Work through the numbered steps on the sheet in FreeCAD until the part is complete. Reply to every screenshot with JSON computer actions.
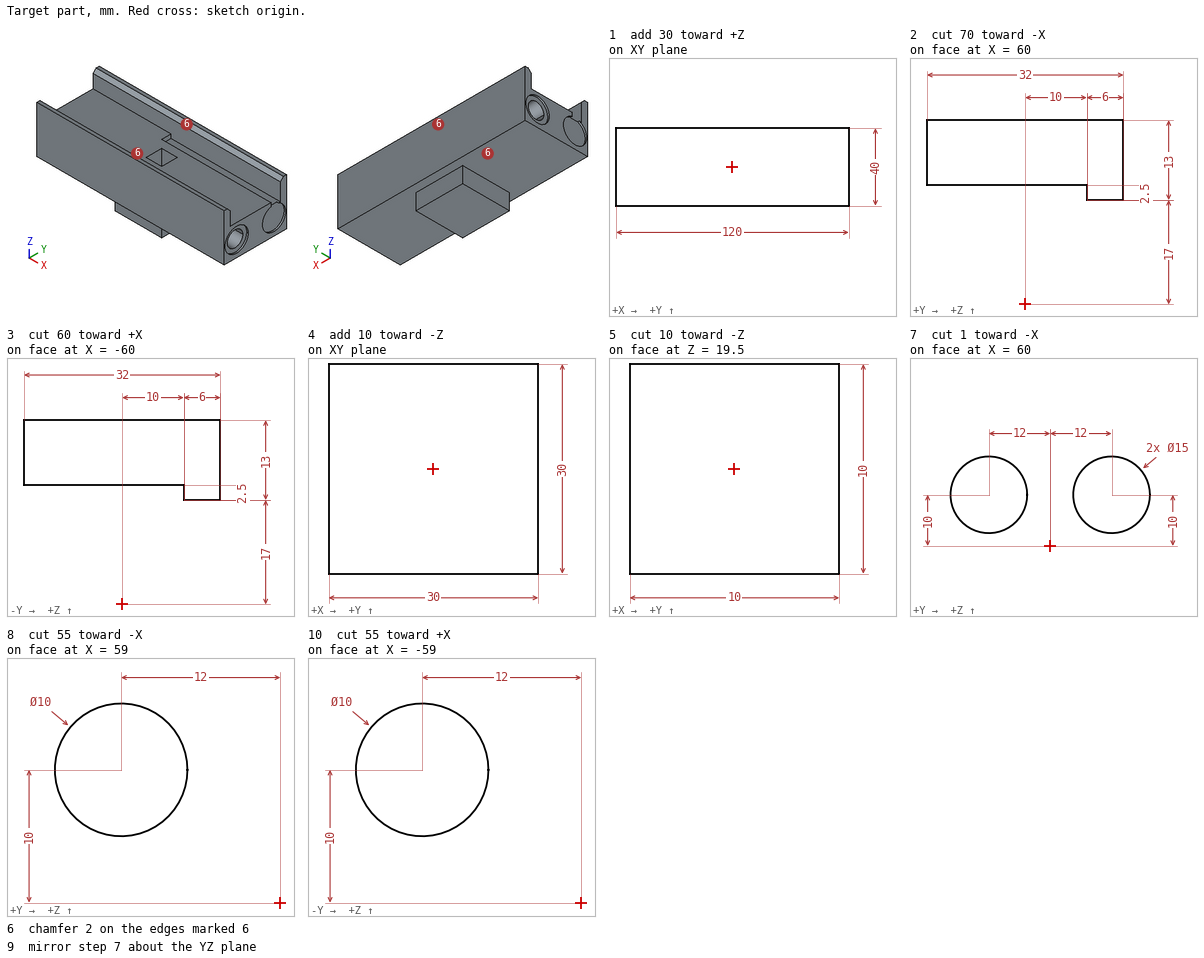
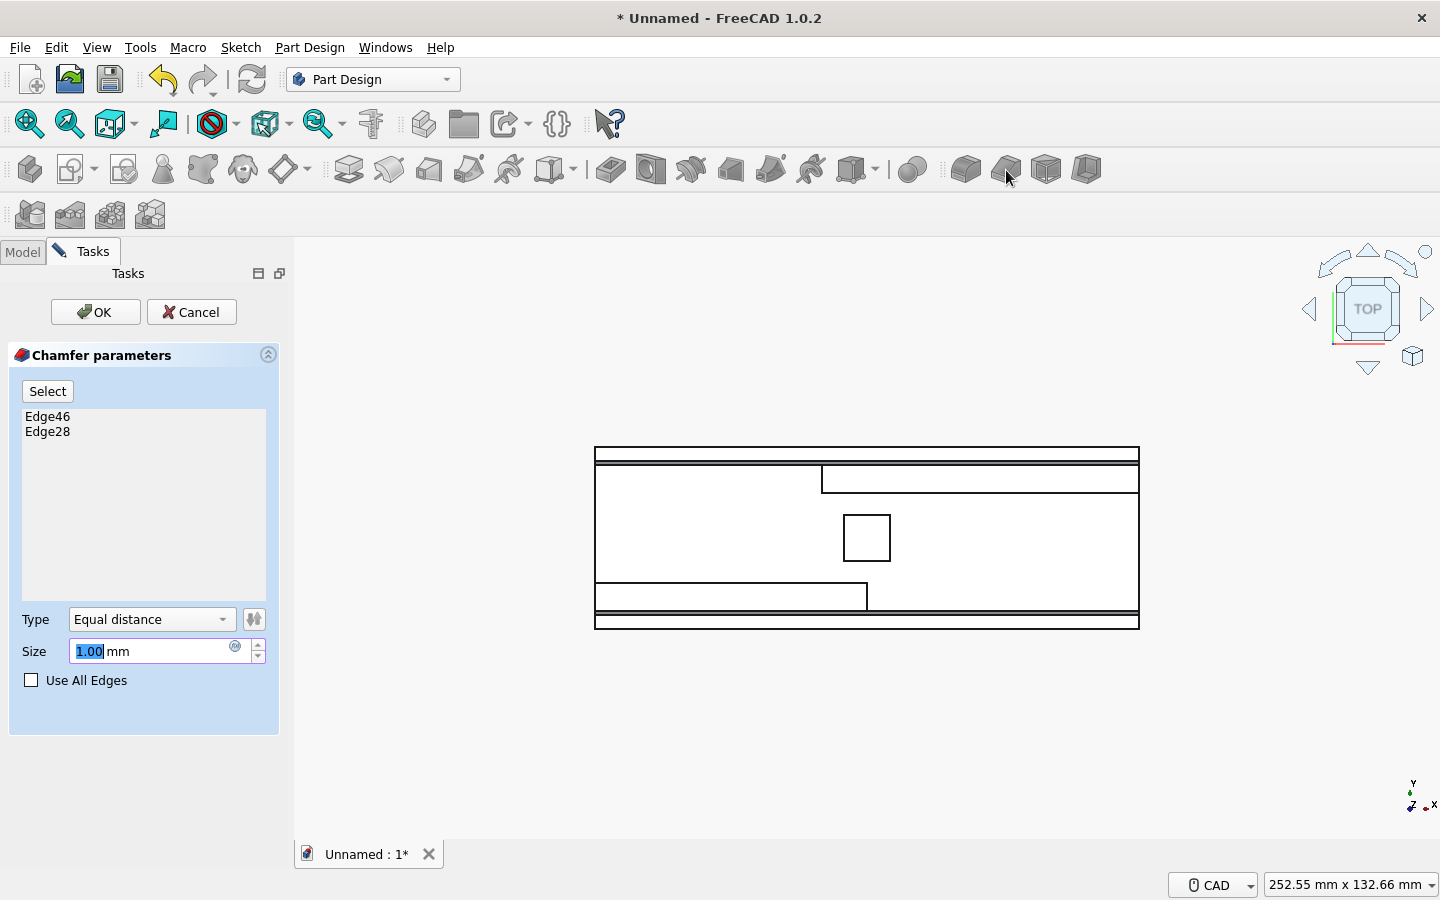
{"action": "type", "text": "2"}
{"action": "key", "text": "Tab"}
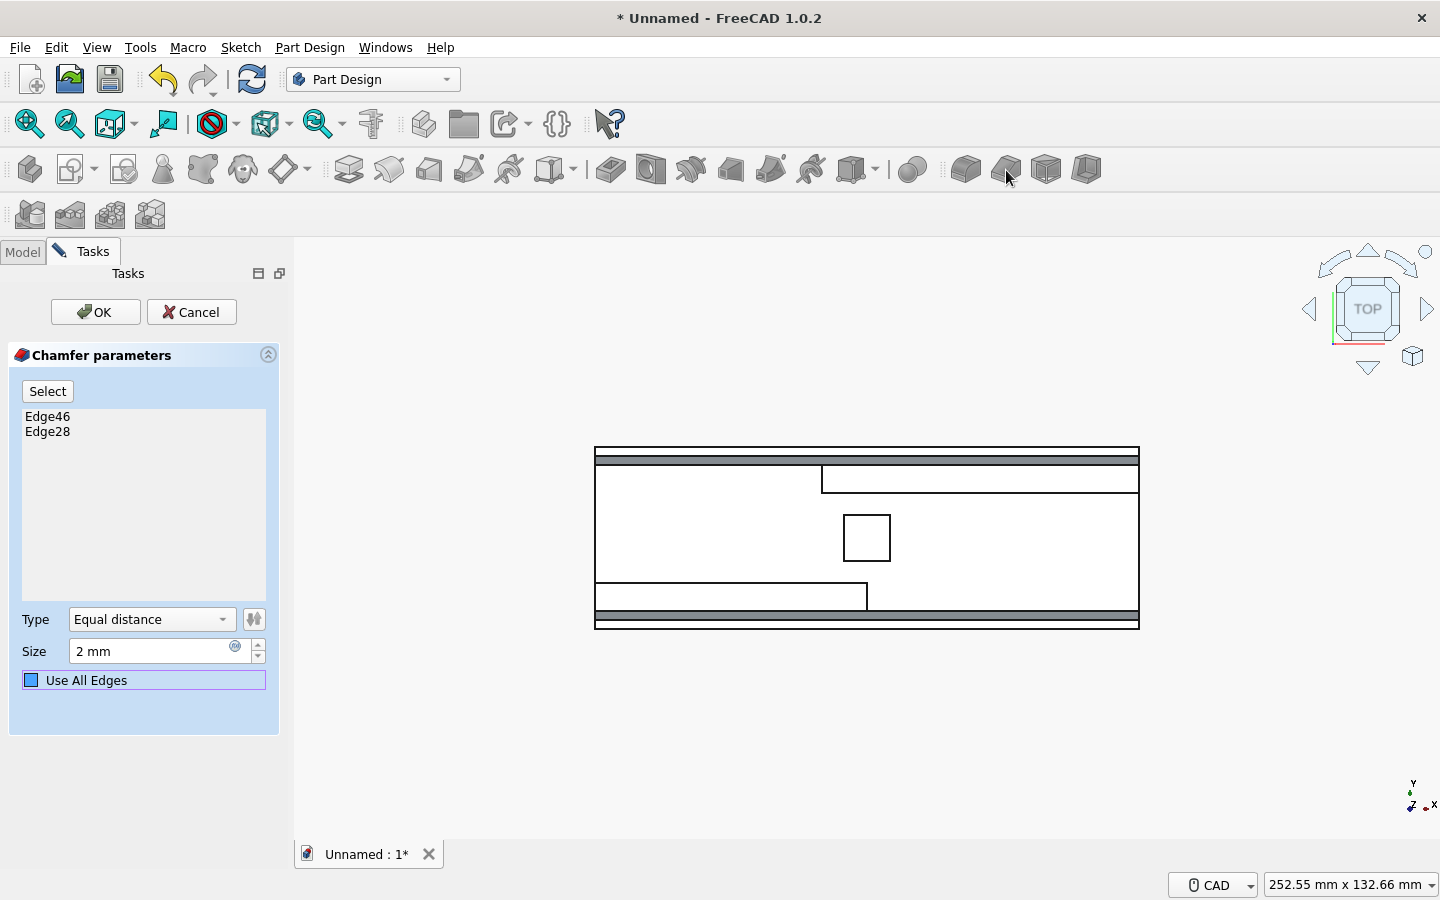
{"action": "left_click", "coordinate": [96, 312]}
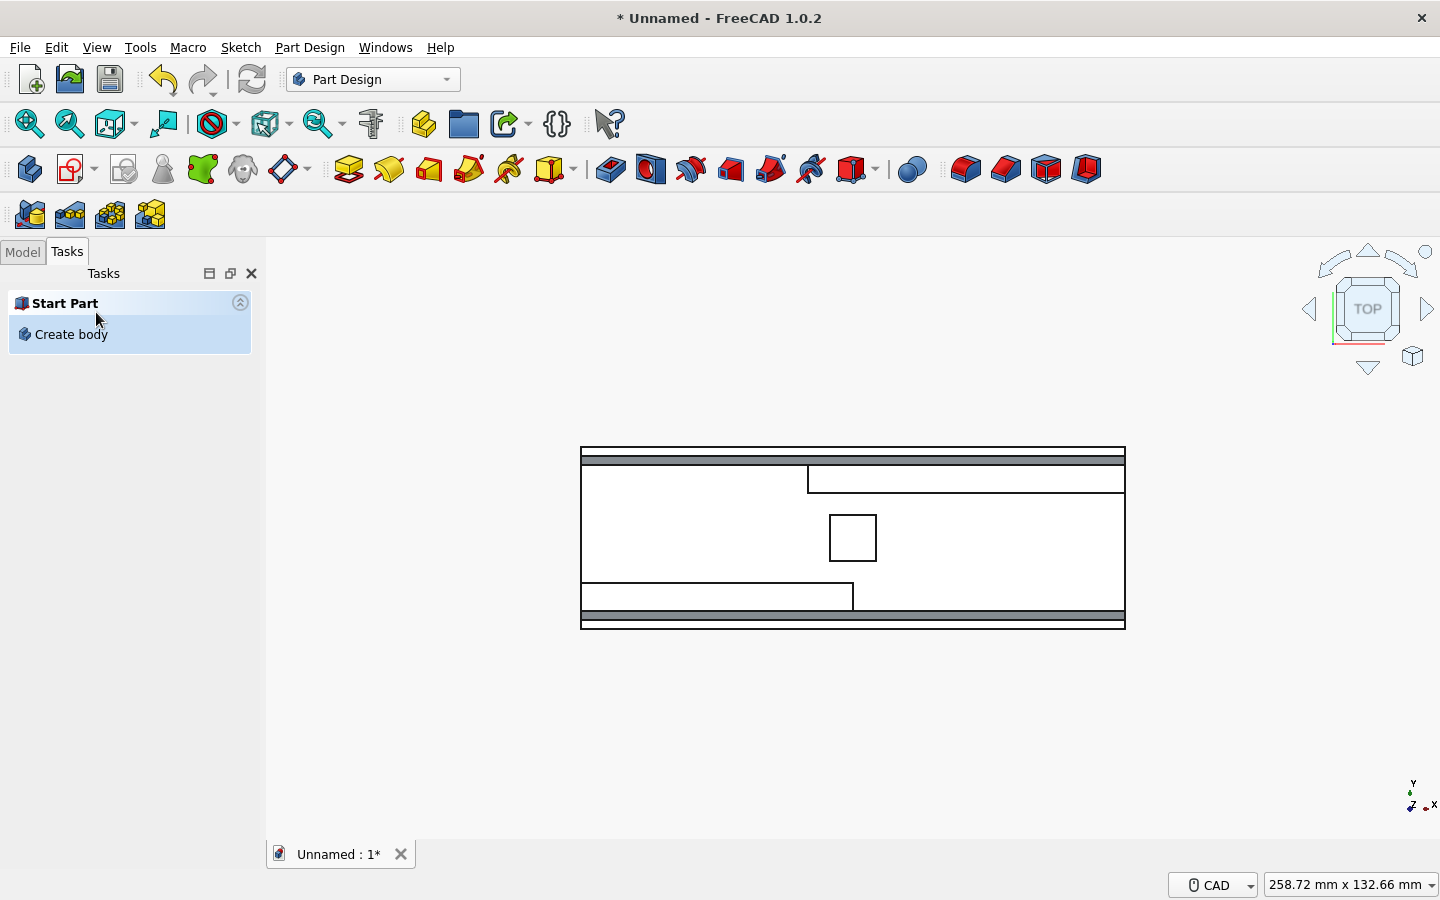
{"action": "key", "text": "0"}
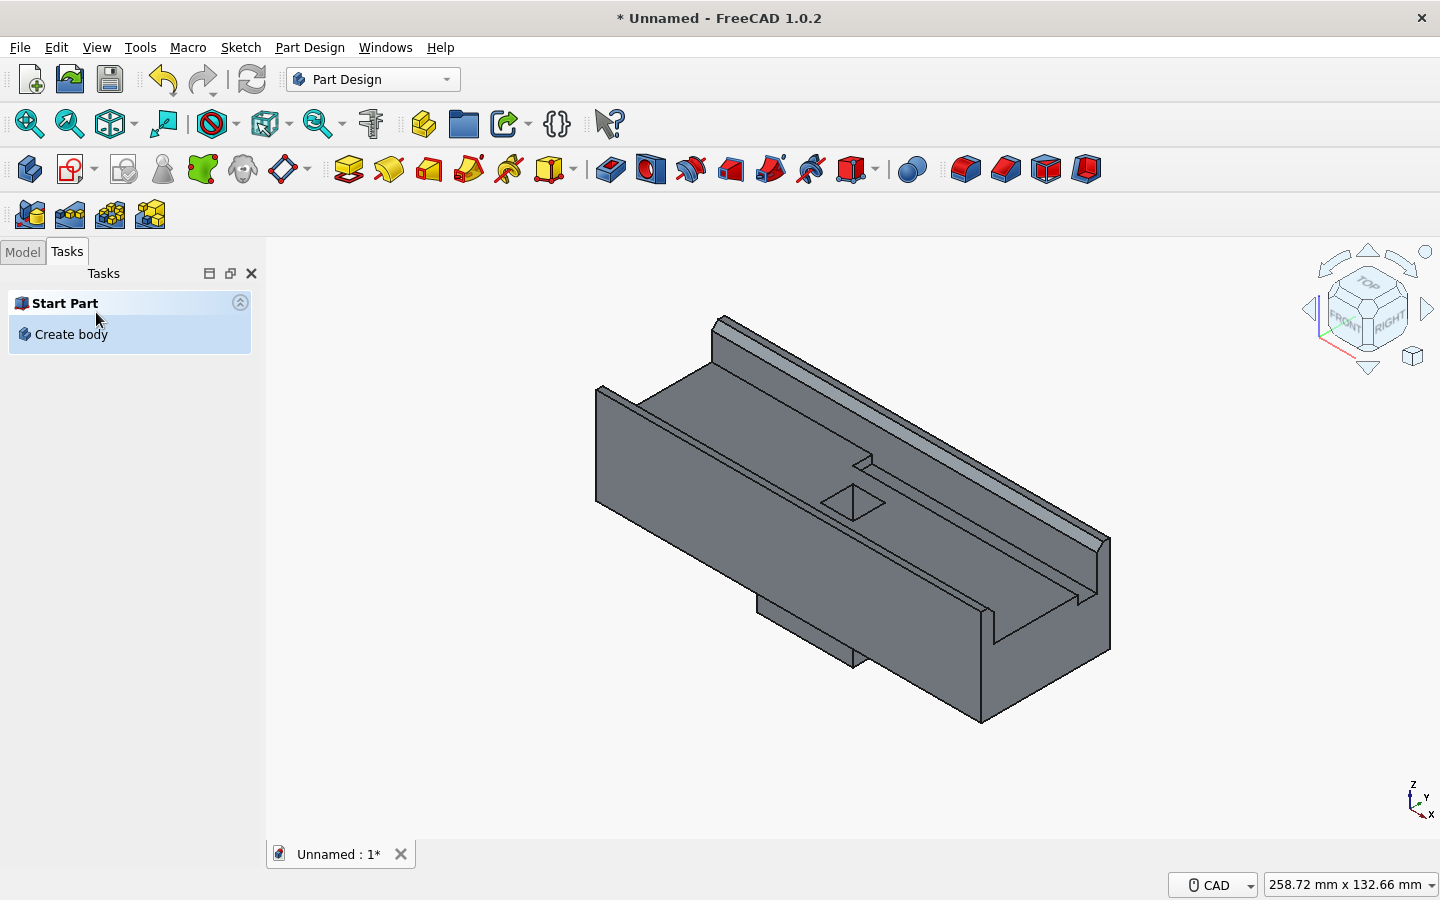
{"action": "left_click", "coordinate": [1046, 646]}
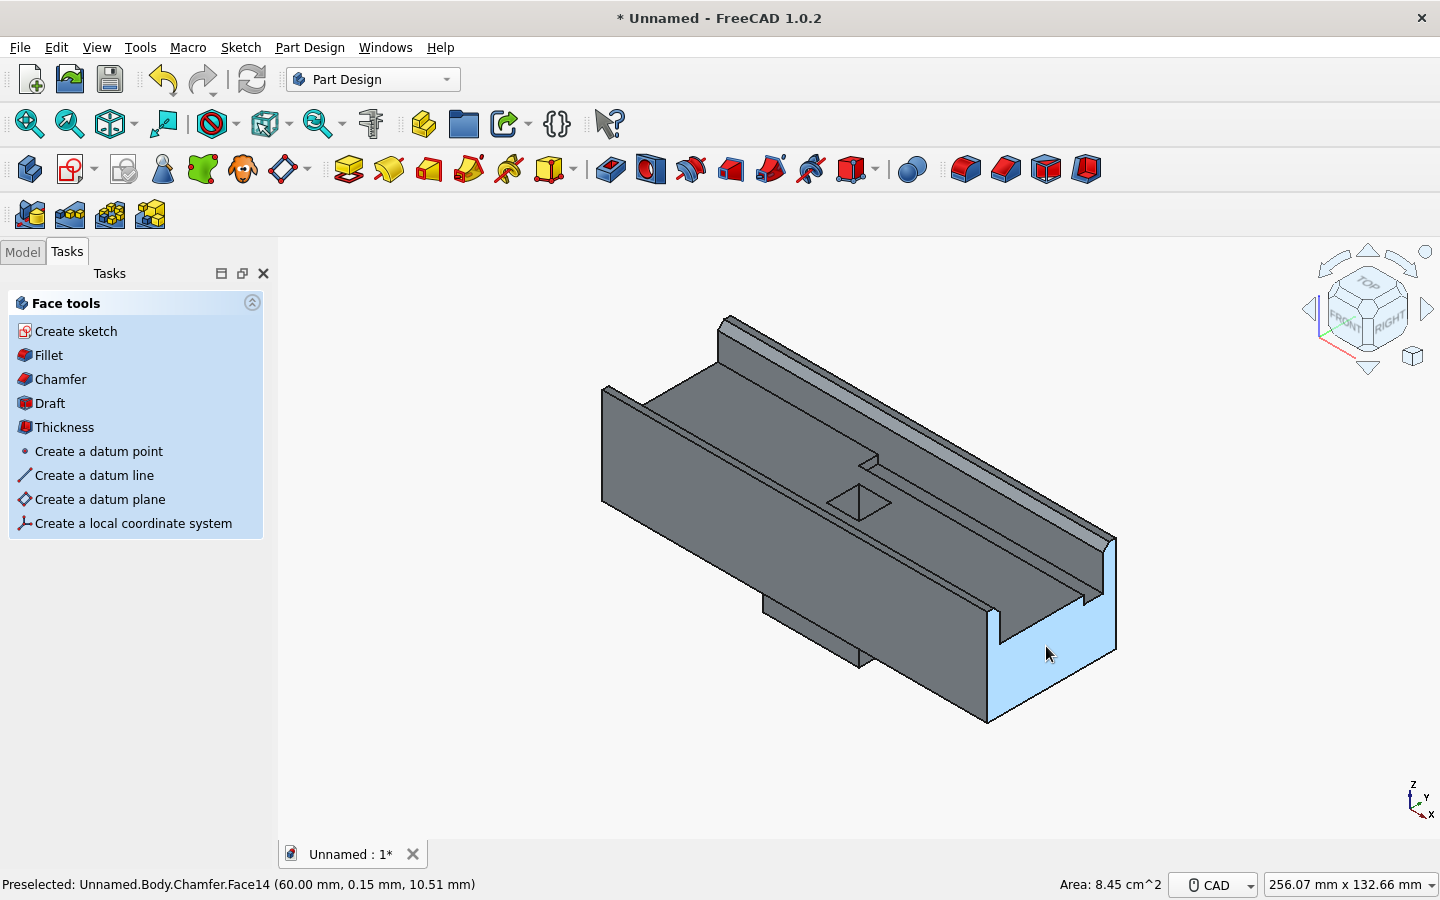
{"action": "left_click", "coordinate": [70, 170]}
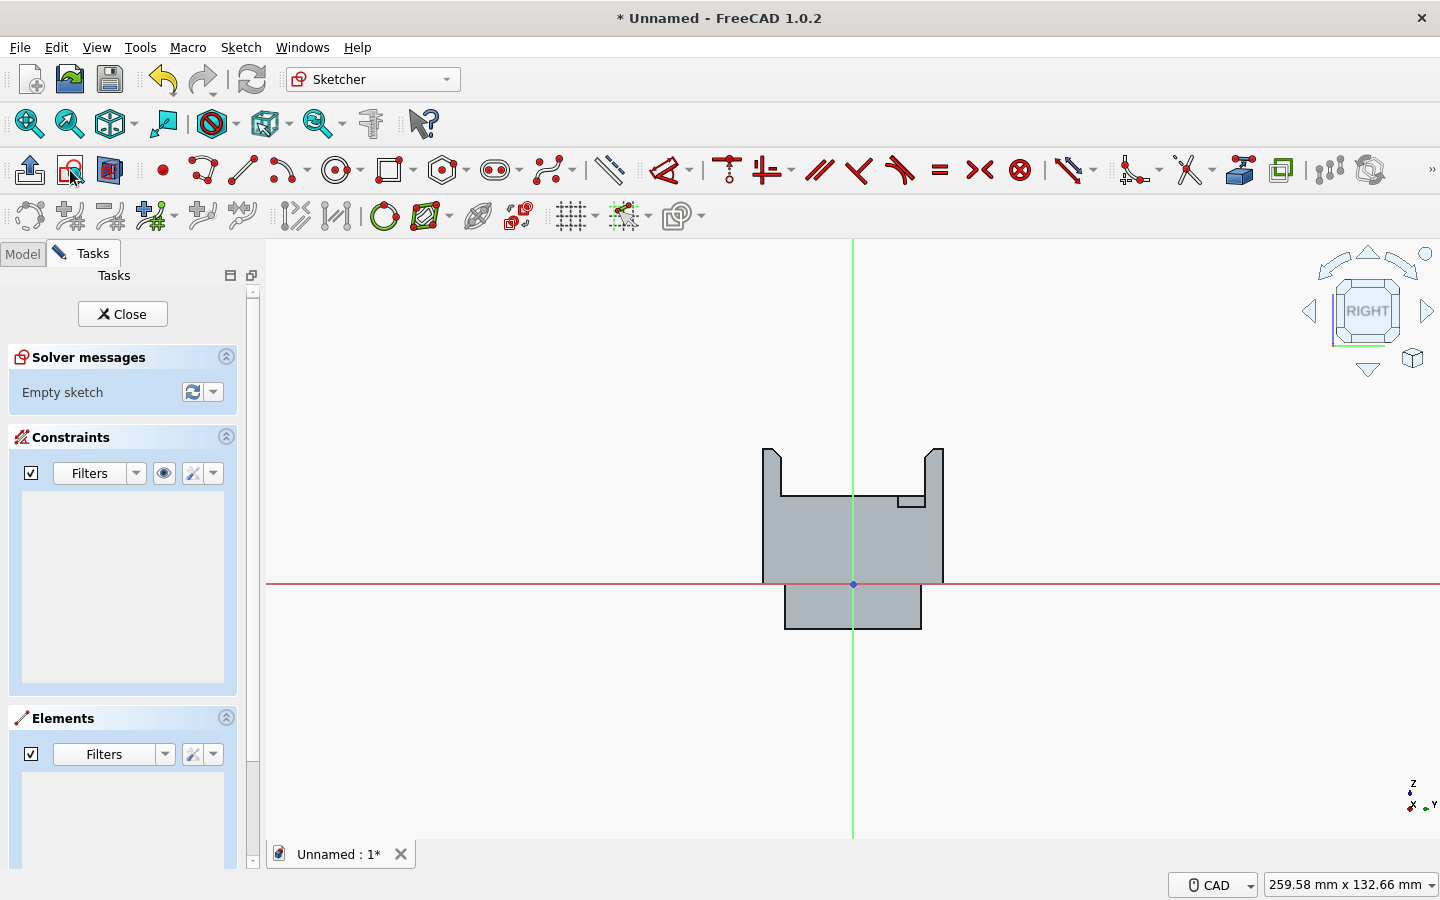
{"action": "scroll", "coordinate": [875, 547], "scroll_direction": "up", "scroll_amount": 7}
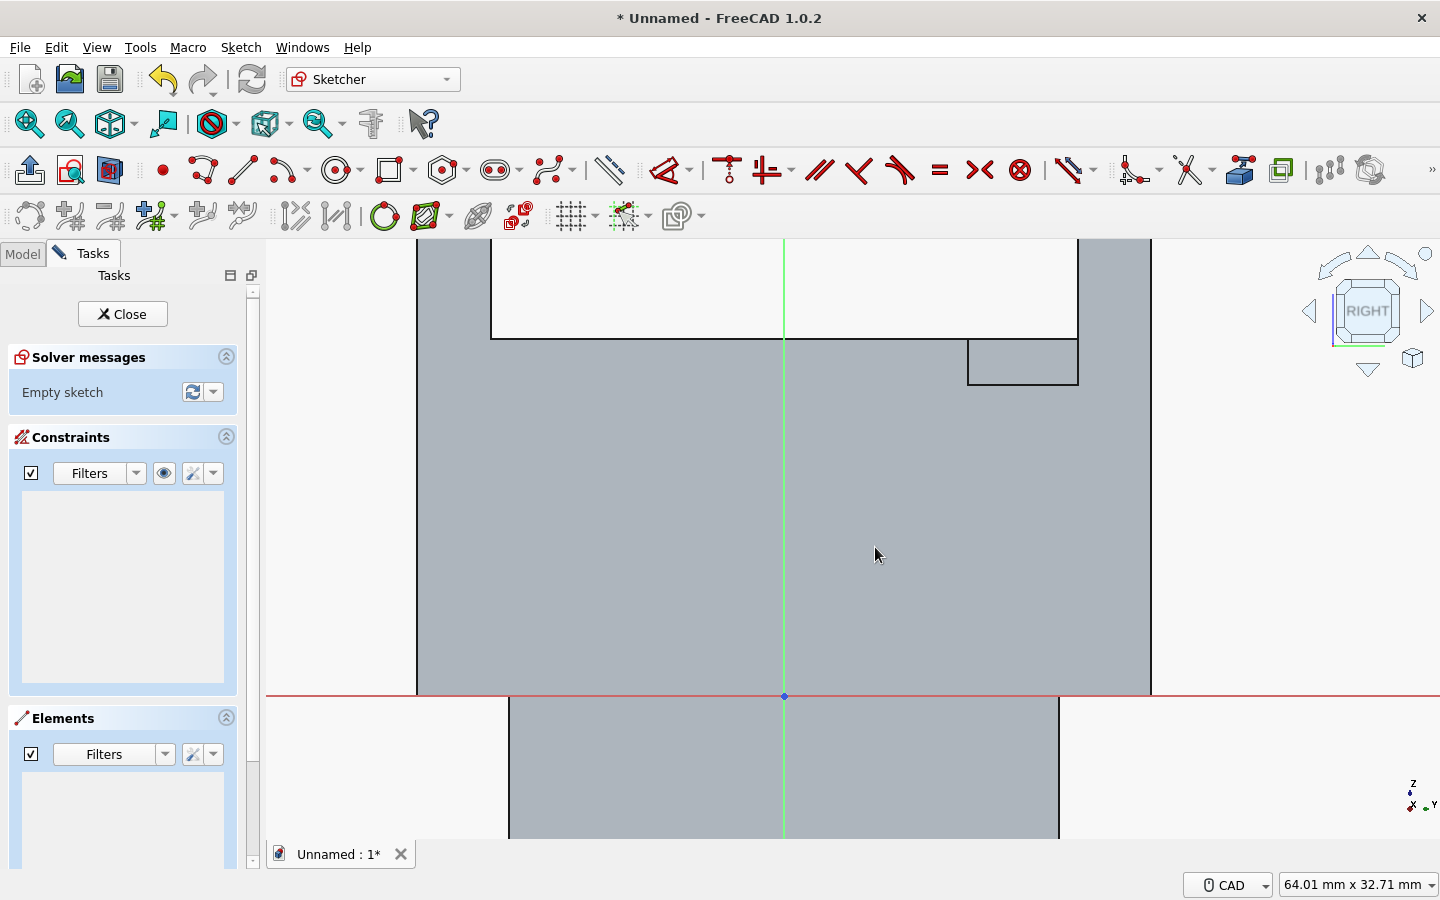
{"action": "left_click", "coordinate": [336, 170]}